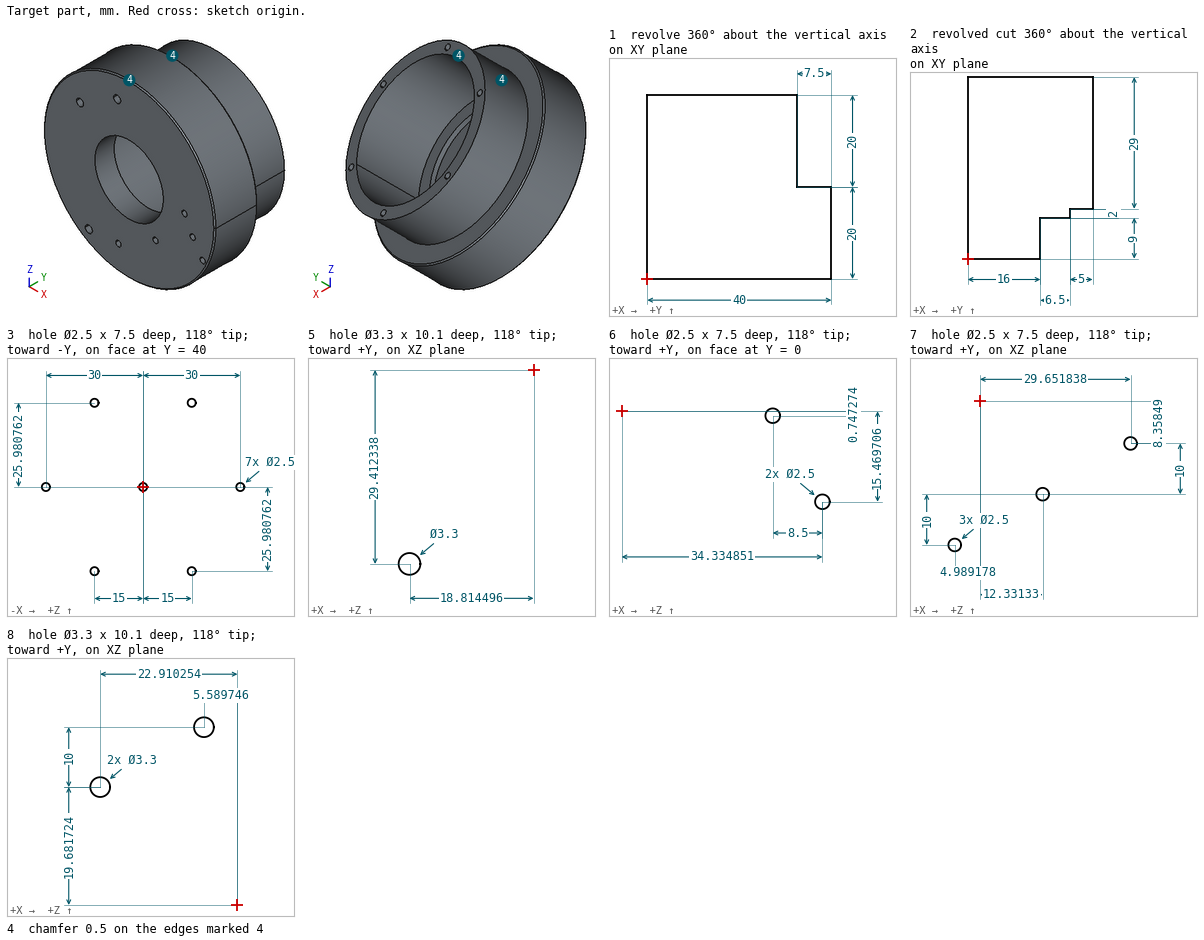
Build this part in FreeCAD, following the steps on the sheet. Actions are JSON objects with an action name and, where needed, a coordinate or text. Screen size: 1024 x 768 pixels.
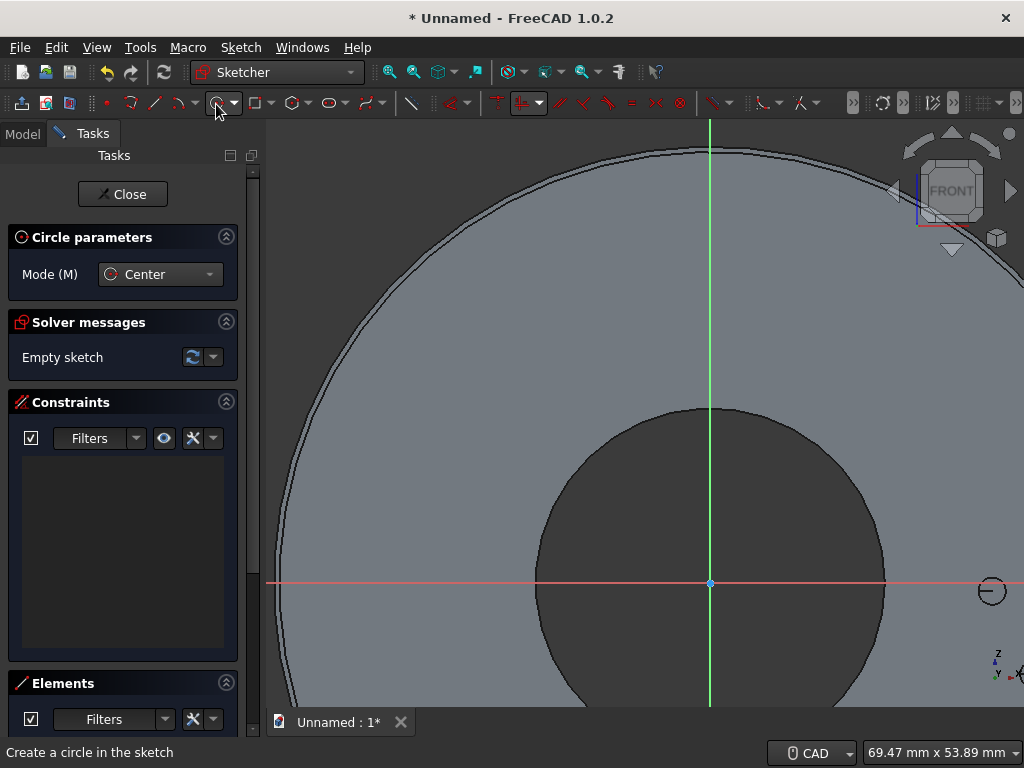
{"action": "scroll", "coordinate": [460, 368], "scroll_direction": "up", "scroll_amount": 2}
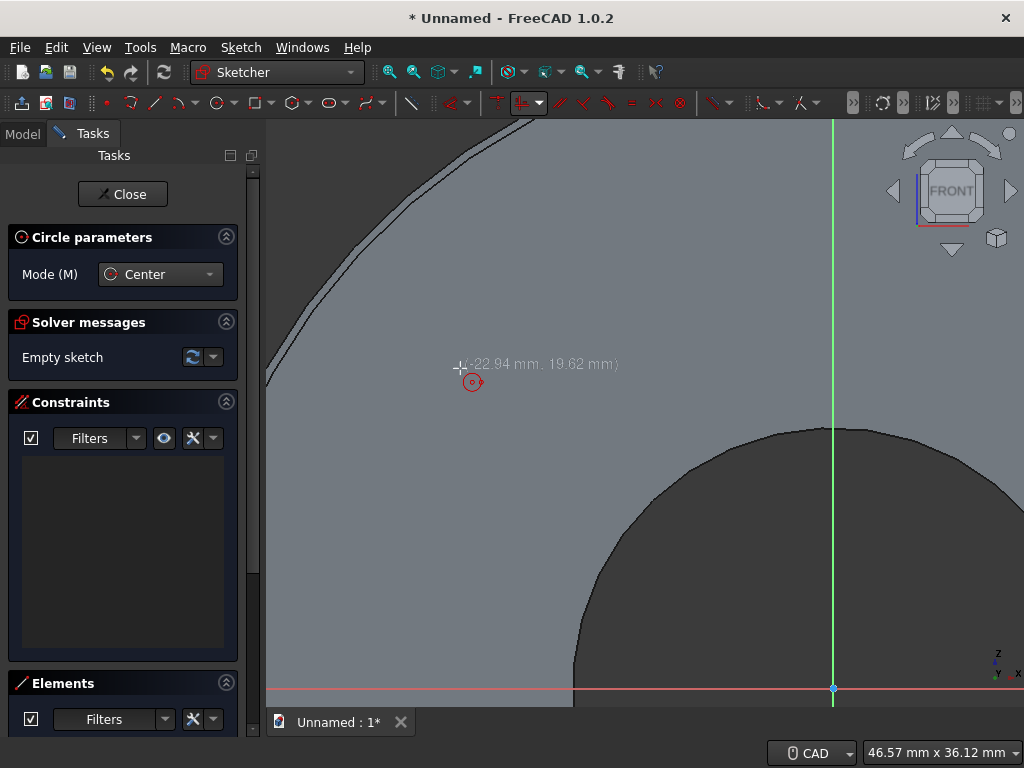
{"action": "left_click", "coordinate": [460, 368]}
{"action": "mouse_move", "coordinate": [479, 349]}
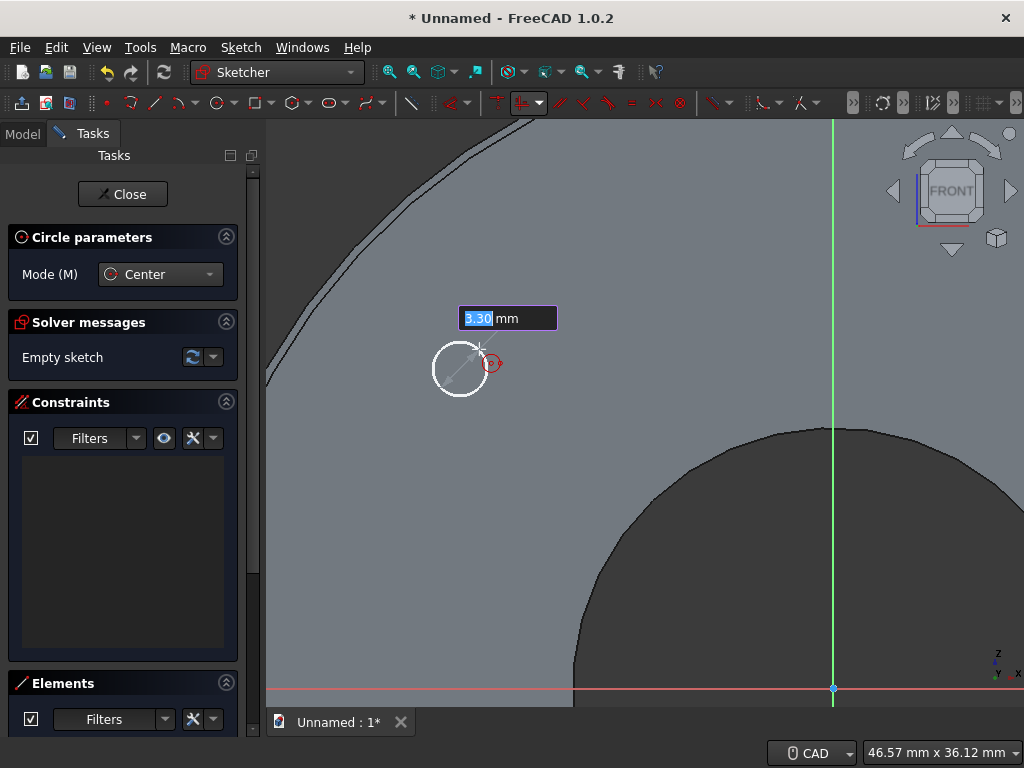
{"action": "type", "text": "3.3"}
{"action": "key", "text": "Return"}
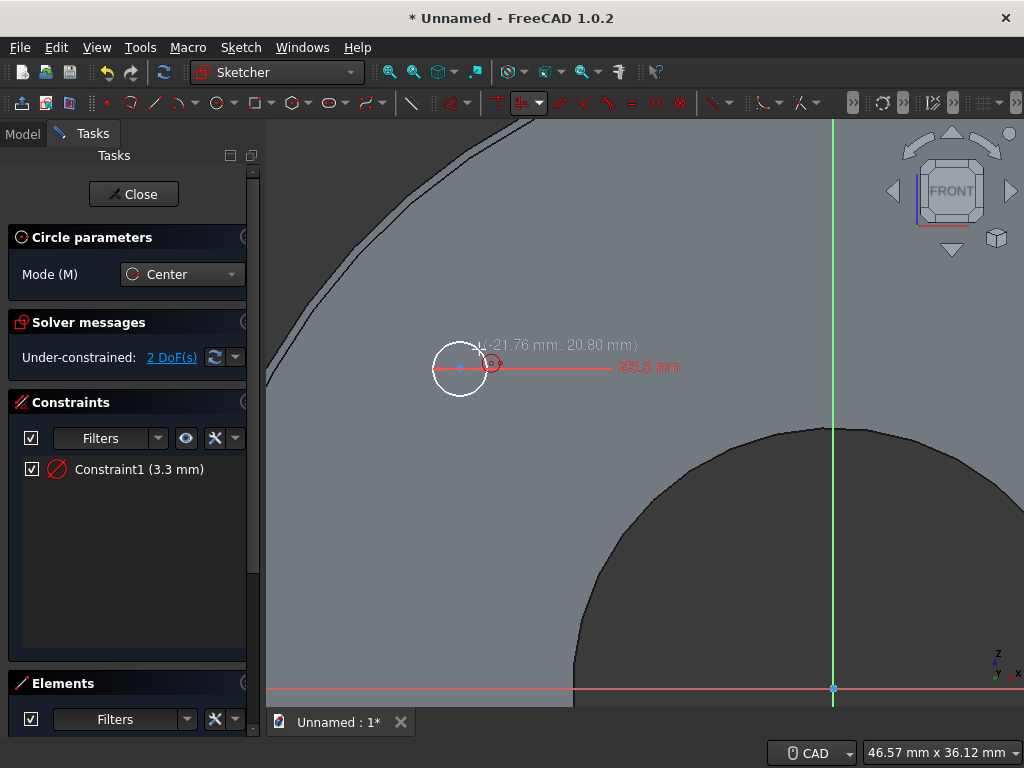
{"action": "left_click", "coordinate": [742, 205]}
{"action": "mouse_move", "coordinate": [761, 186]}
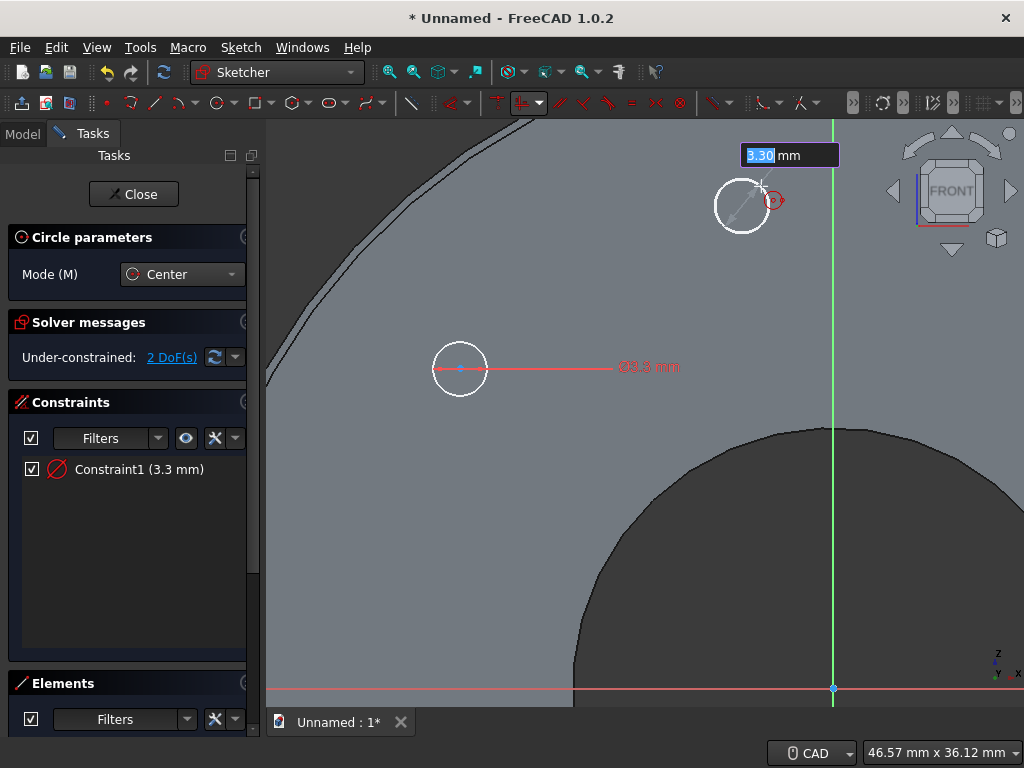
{"action": "type", "text": "3.3"}
{"action": "key", "text": "Return"}
{"action": "key", "text": "Escape"}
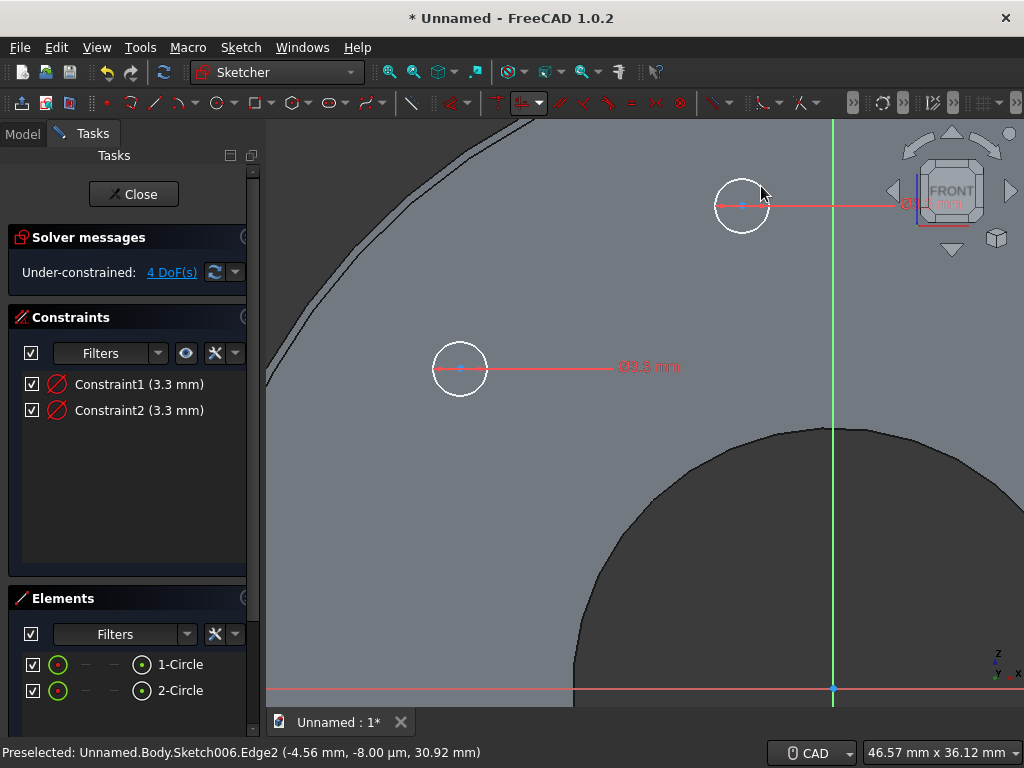
{"action": "left_click", "coordinate": [450, 104]}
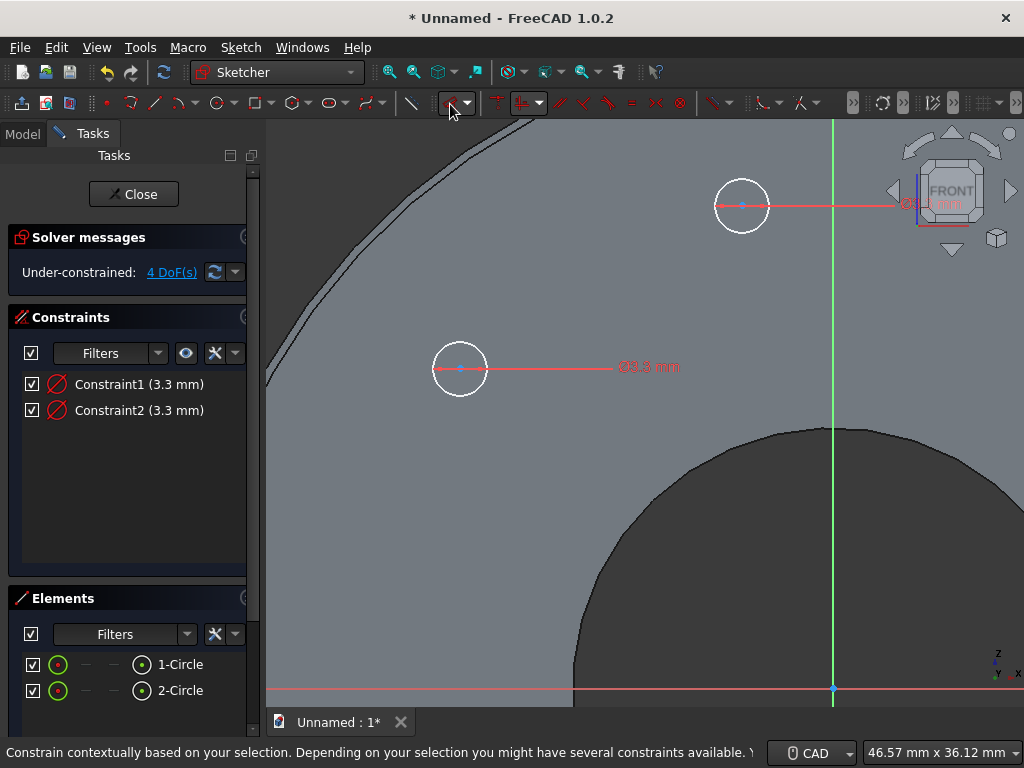
{"action": "left_click", "coordinate": [460, 369]}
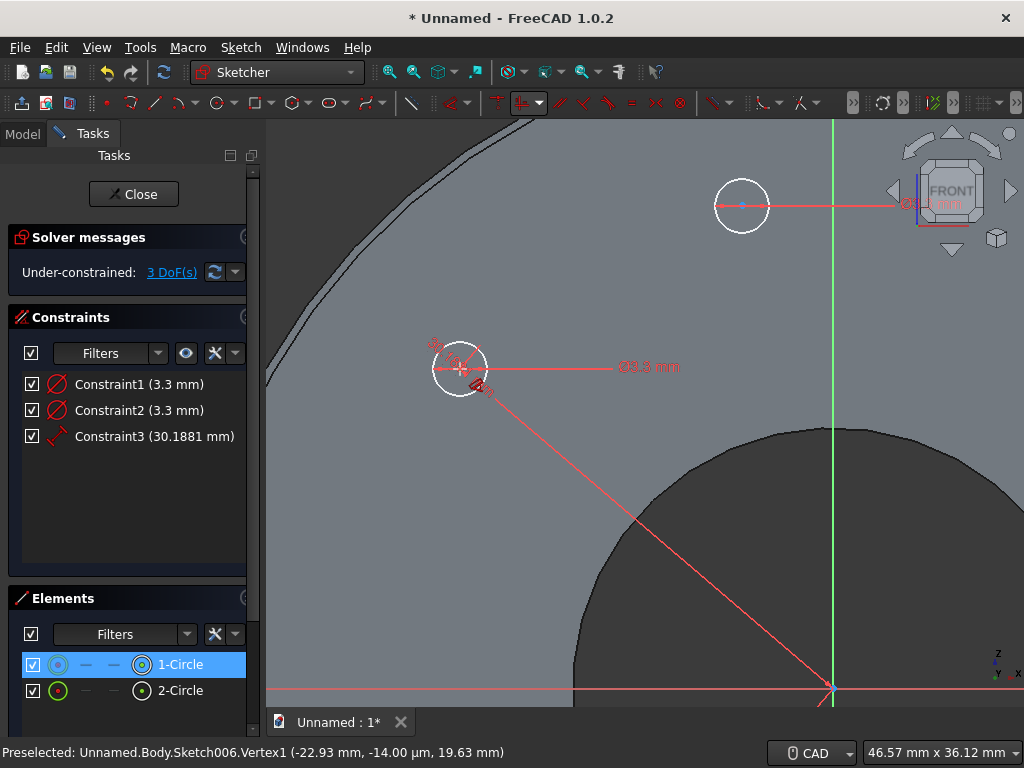
{"action": "left_click", "coordinate": [742, 206]}
{"action": "left_click", "coordinate": [426, 288]}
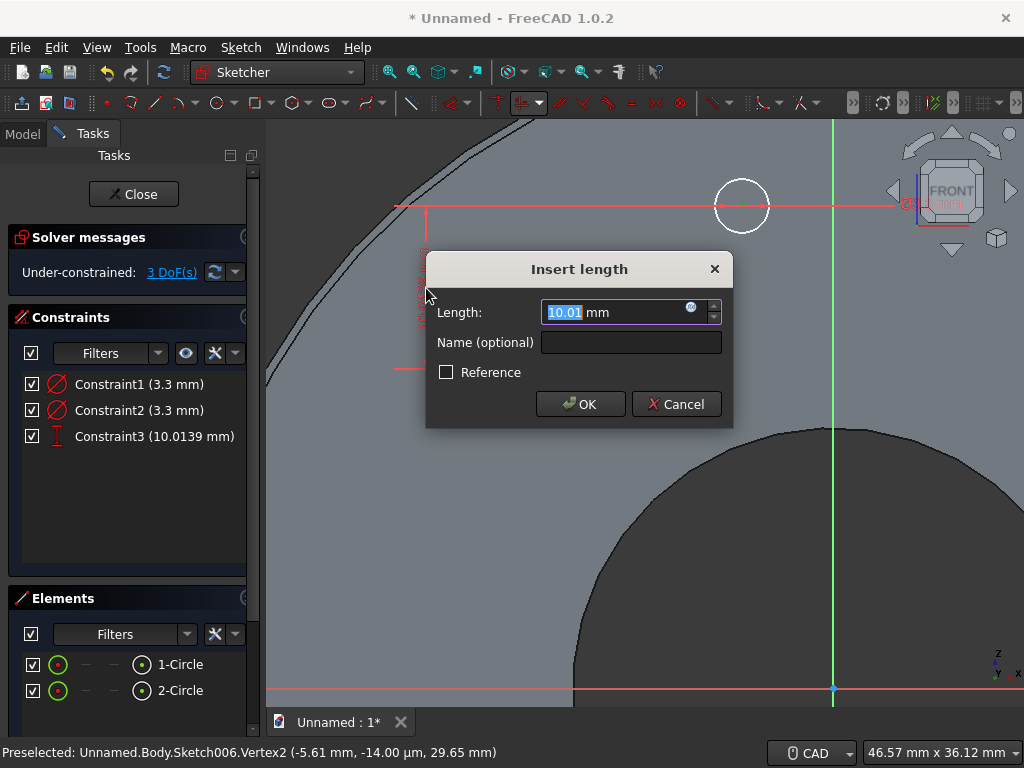
{"action": "type", "text": "10"}
{"action": "key", "text": "Return"}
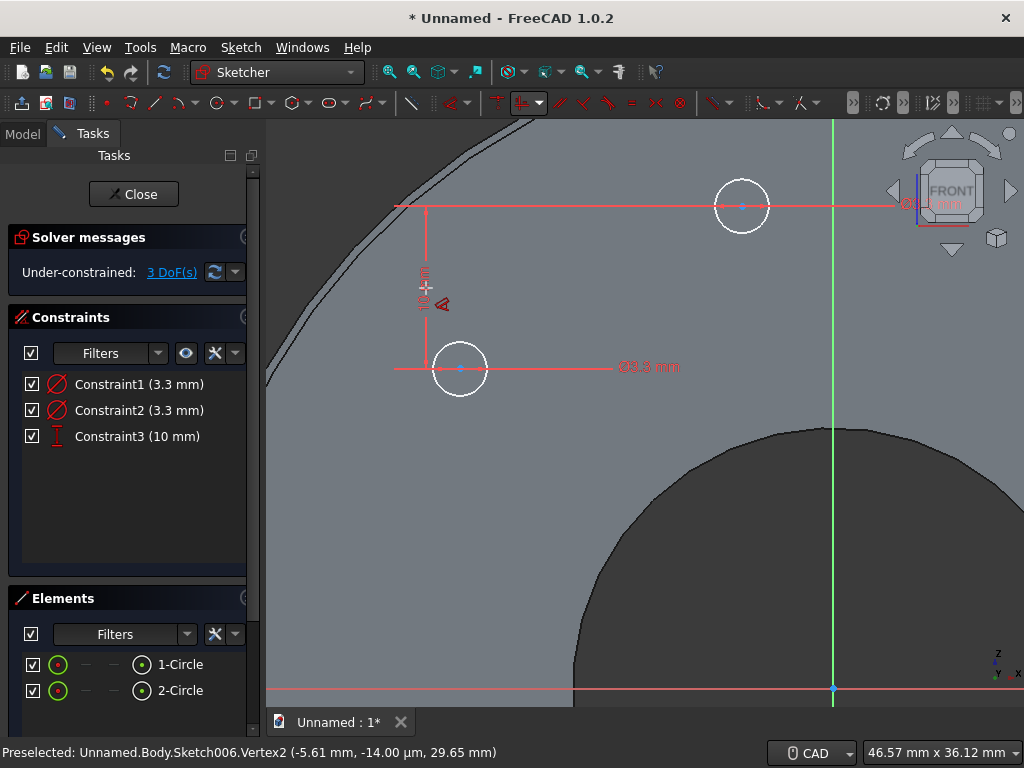
{"action": "left_click", "coordinate": [742, 206]}
{"action": "left_click", "coordinate": [788, 172]}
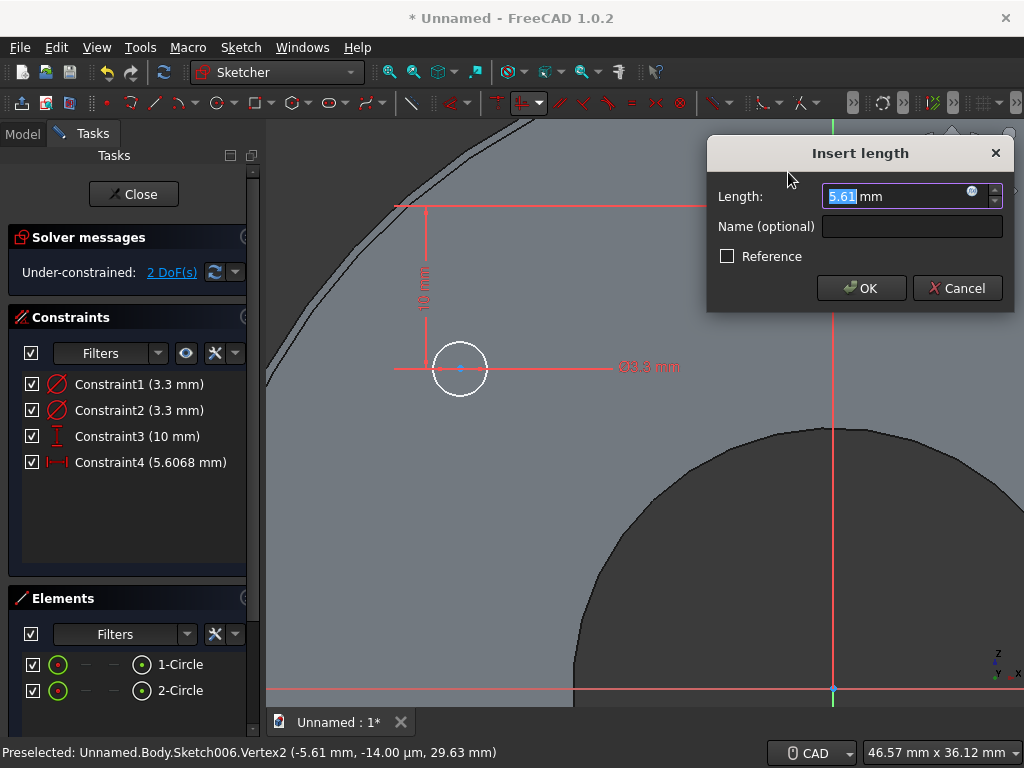
{"action": "type", "text": "5.589746"}
{"action": "key", "text": "Return"}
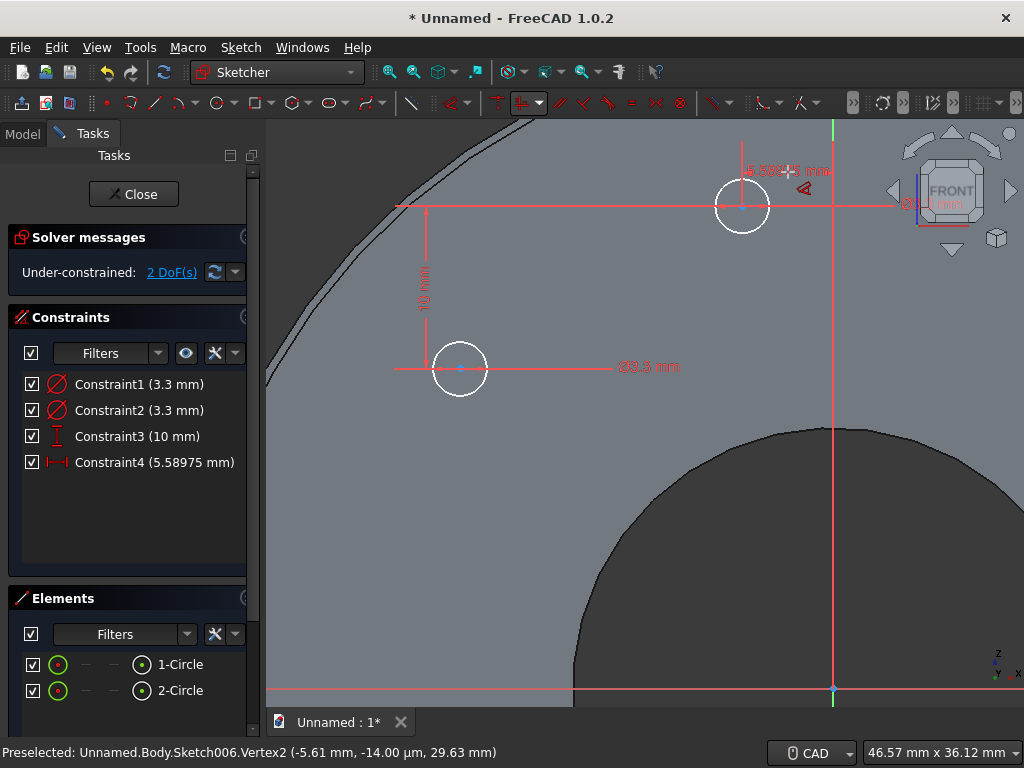
{"action": "left_click", "coordinate": [460, 369]}
{"action": "left_click", "coordinate": [647, 335]}